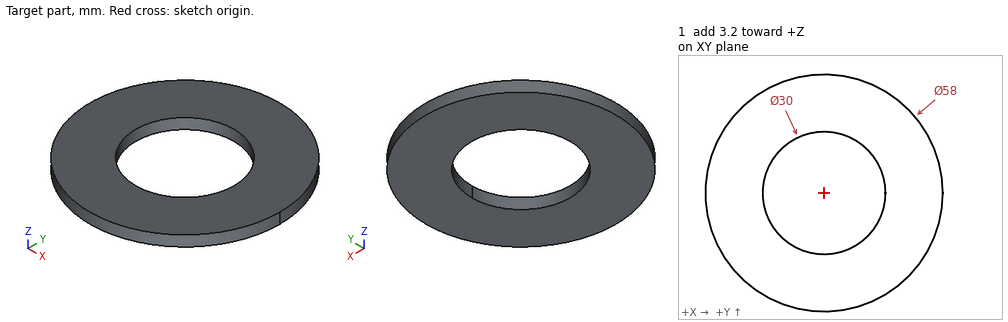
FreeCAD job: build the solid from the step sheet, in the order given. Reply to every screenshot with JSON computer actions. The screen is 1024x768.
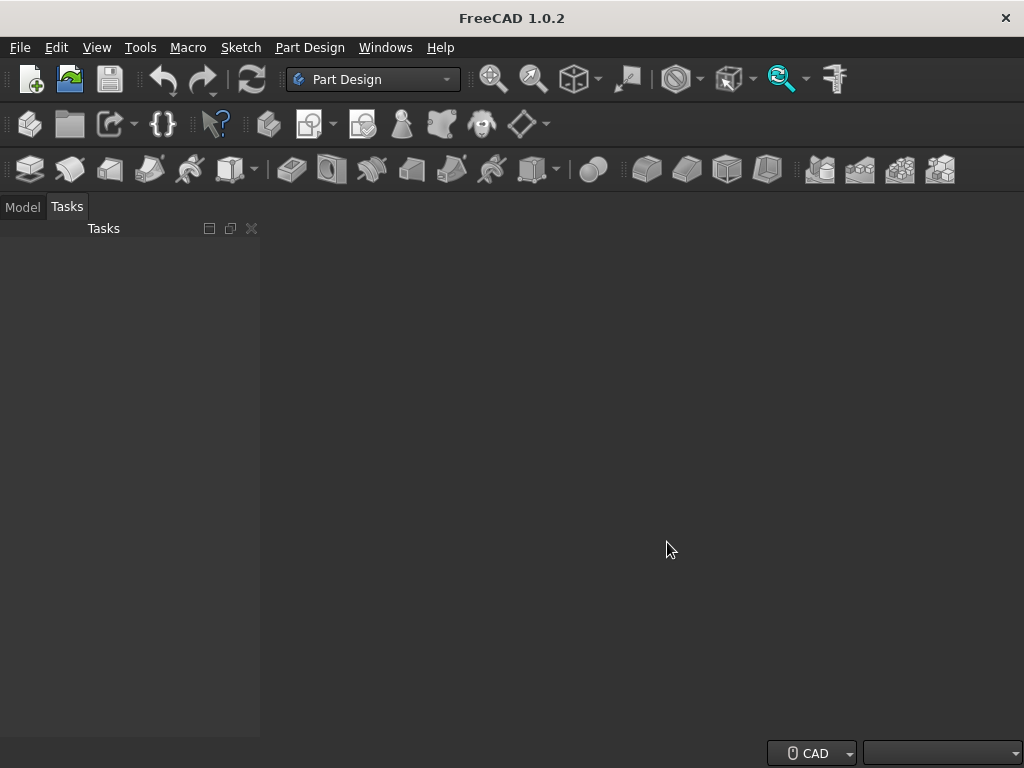
{"action": "left_click", "coordinate": [30, 80]}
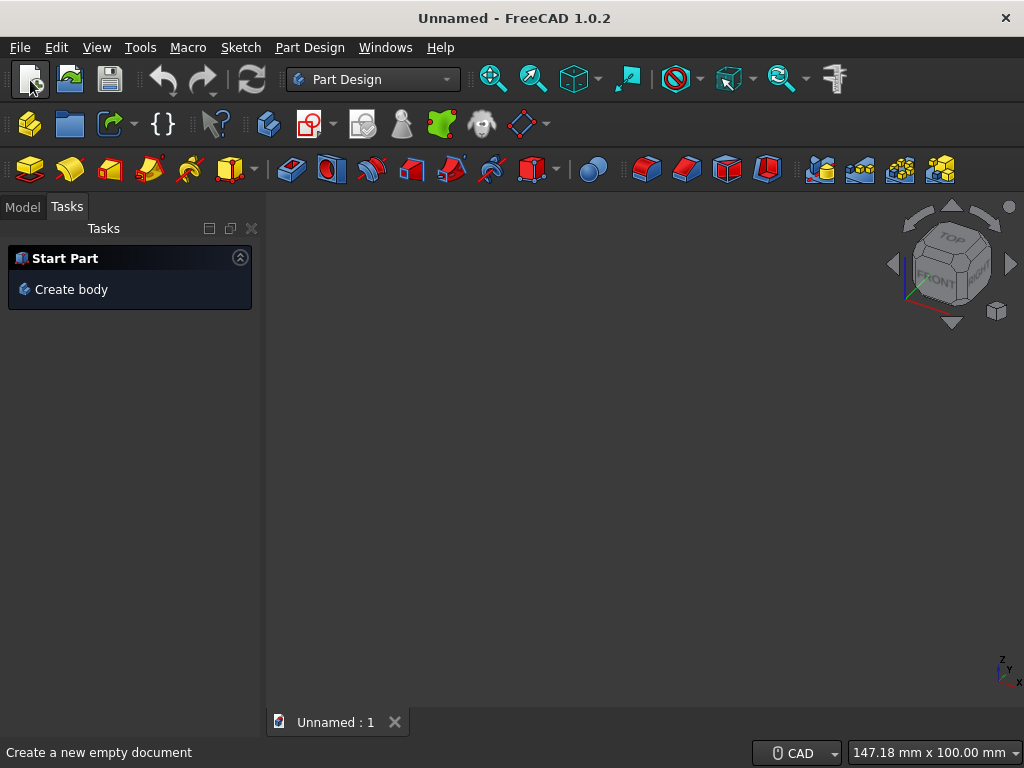
{"action": "left_click", "coordinate": [310, 124]}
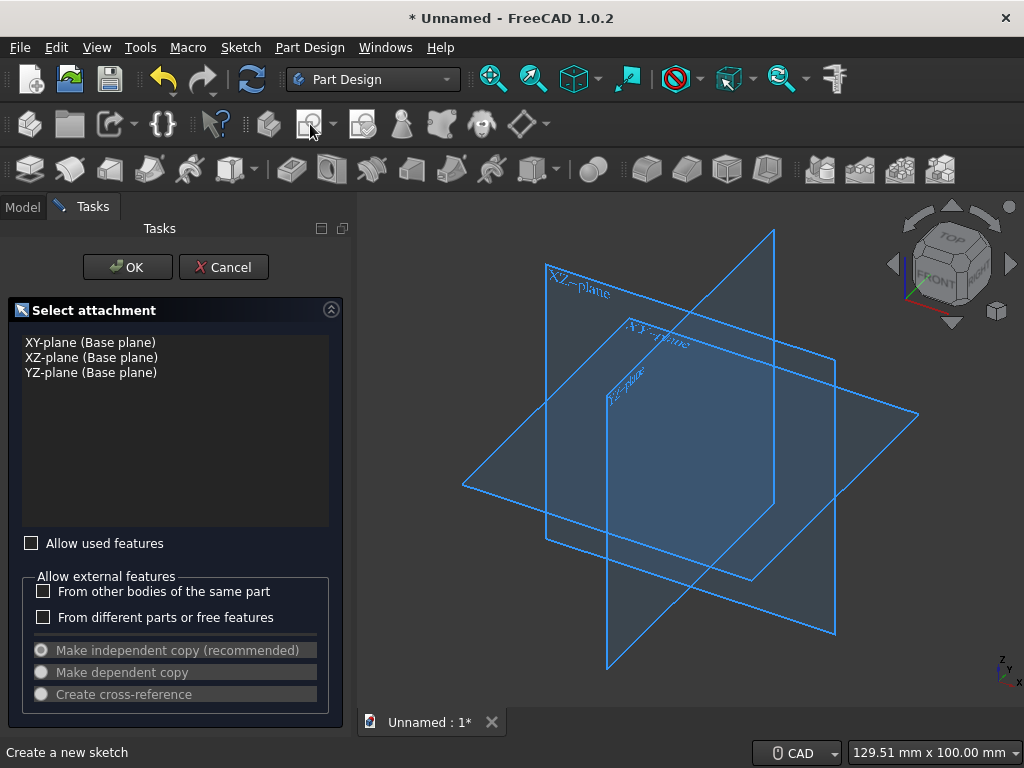
{"action": "left_click", "coordinate": [82, 342]}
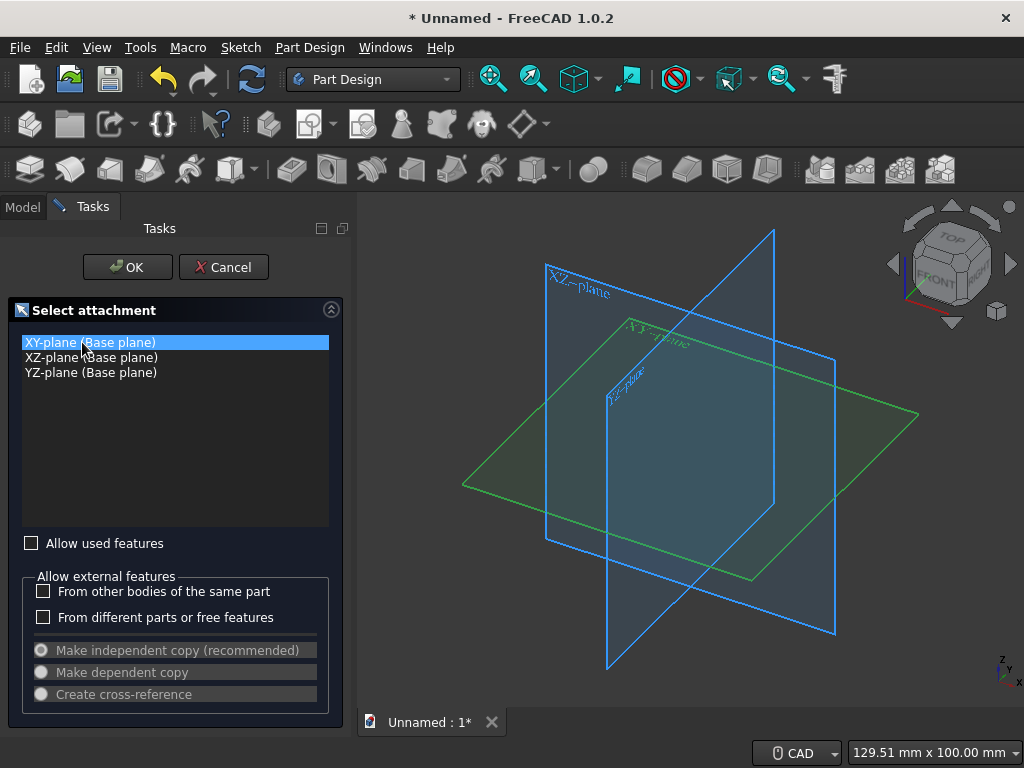
{"action": "left_click", "coordinate": [128, 267]}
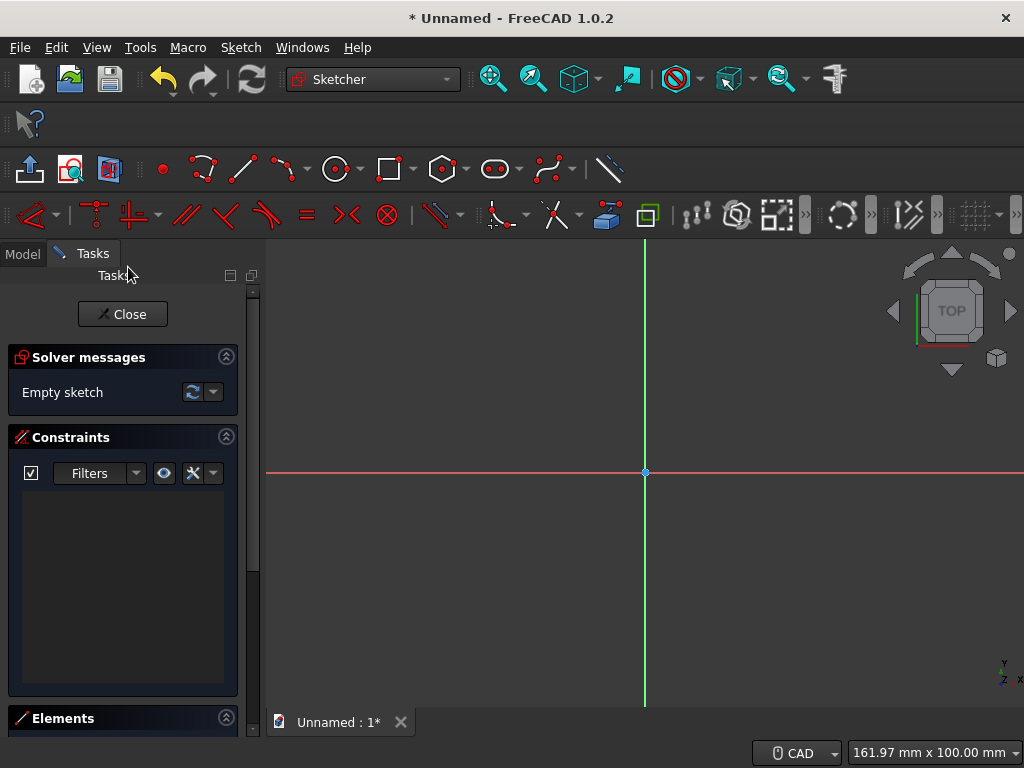
{"action": "left_click", "coordinate": [336, 170]}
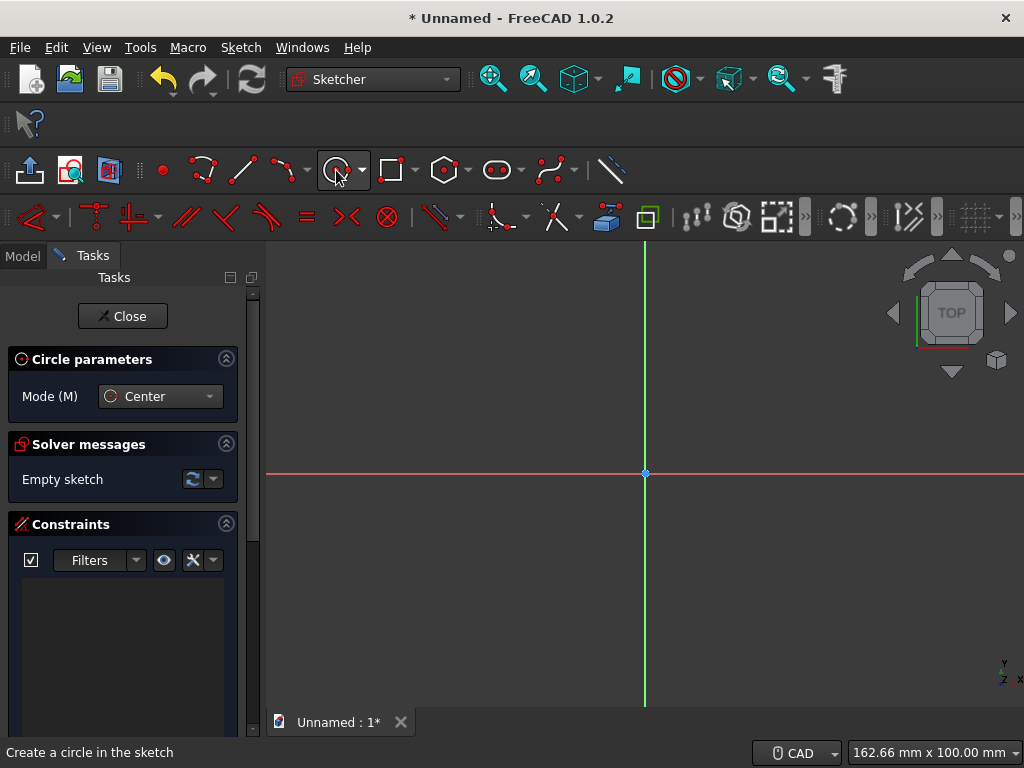
{"action": "left_click", "coordinate": [645, 474]}
{"action": "left_click", "coordinate": [741, 378]}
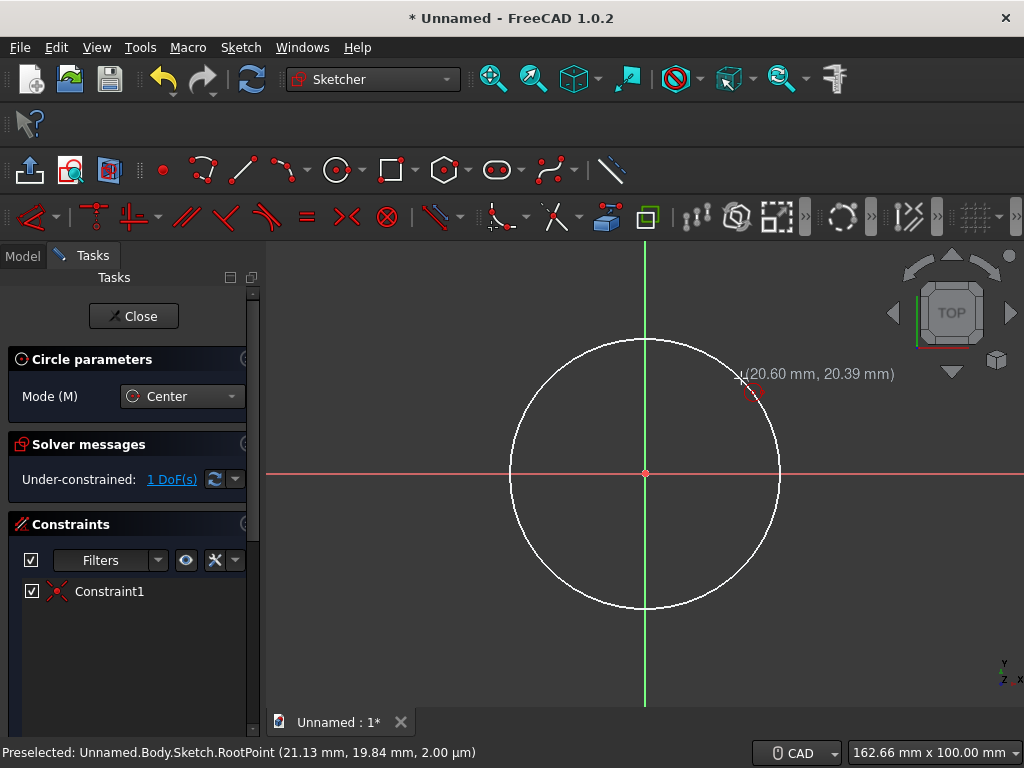
{"action": "left_click", "coordinate": [645, 474]}
{"action": "left_click", "coordinate": [694, 425]}
{"action": "key", "text": "Escape"}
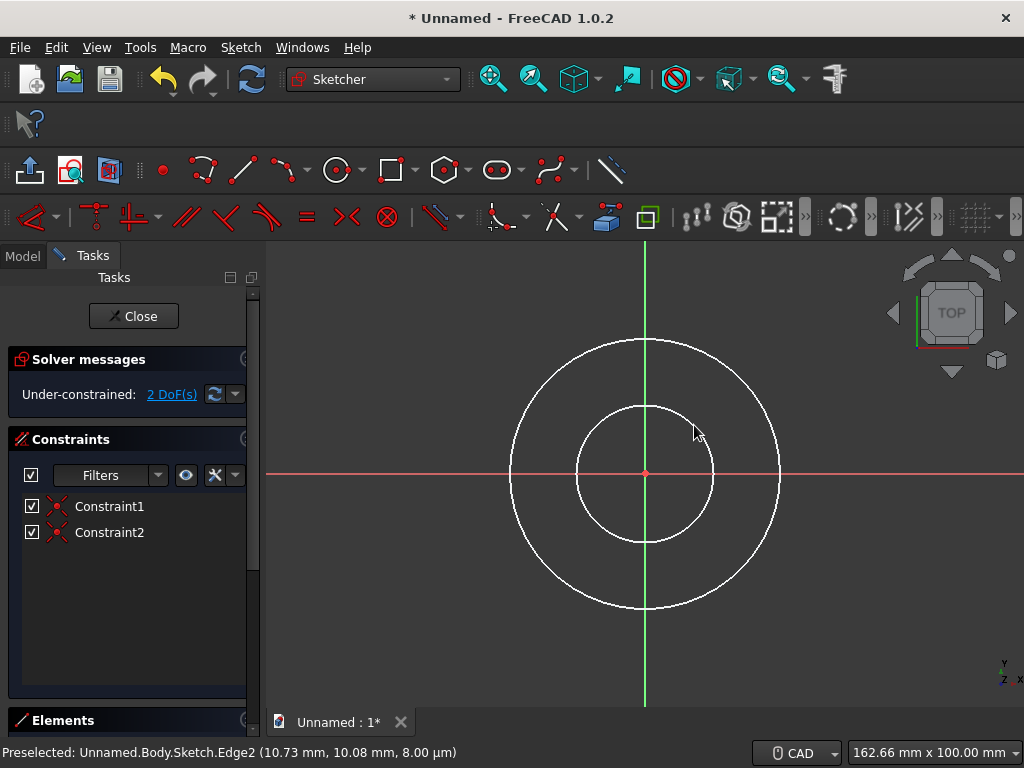
{"action": "left_click", "coordinate": [32, 218]}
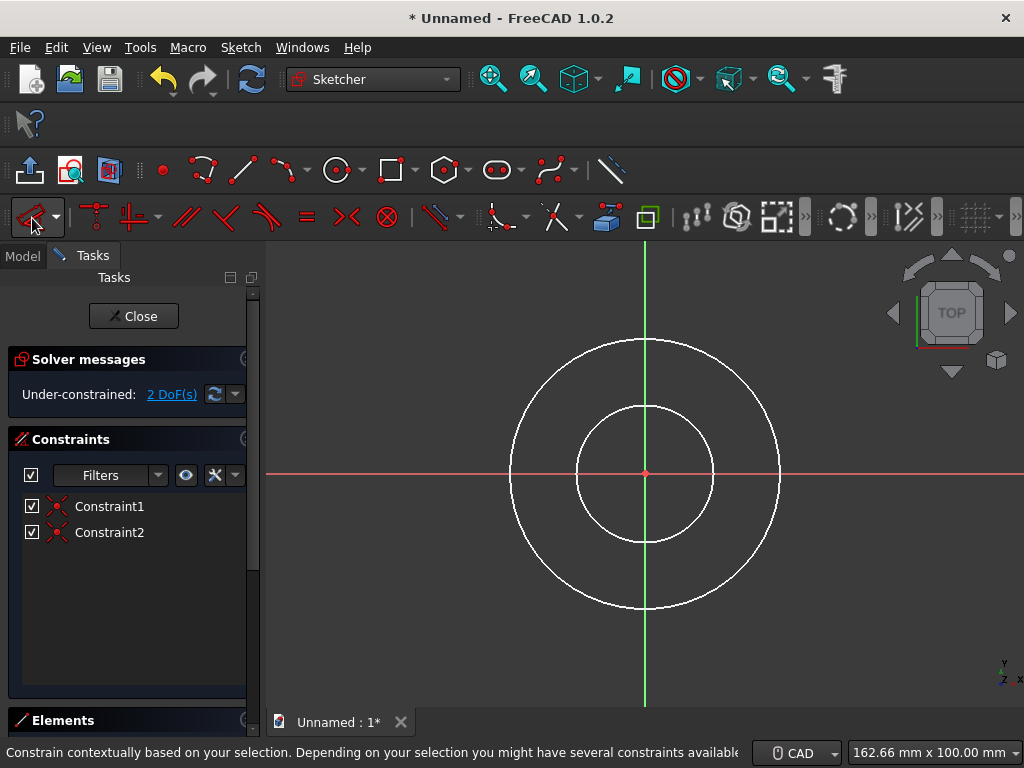
{"action": "left_click", "coordinate": [740, 378]}
{"action": "left_click", "coordinate": [763, 355]}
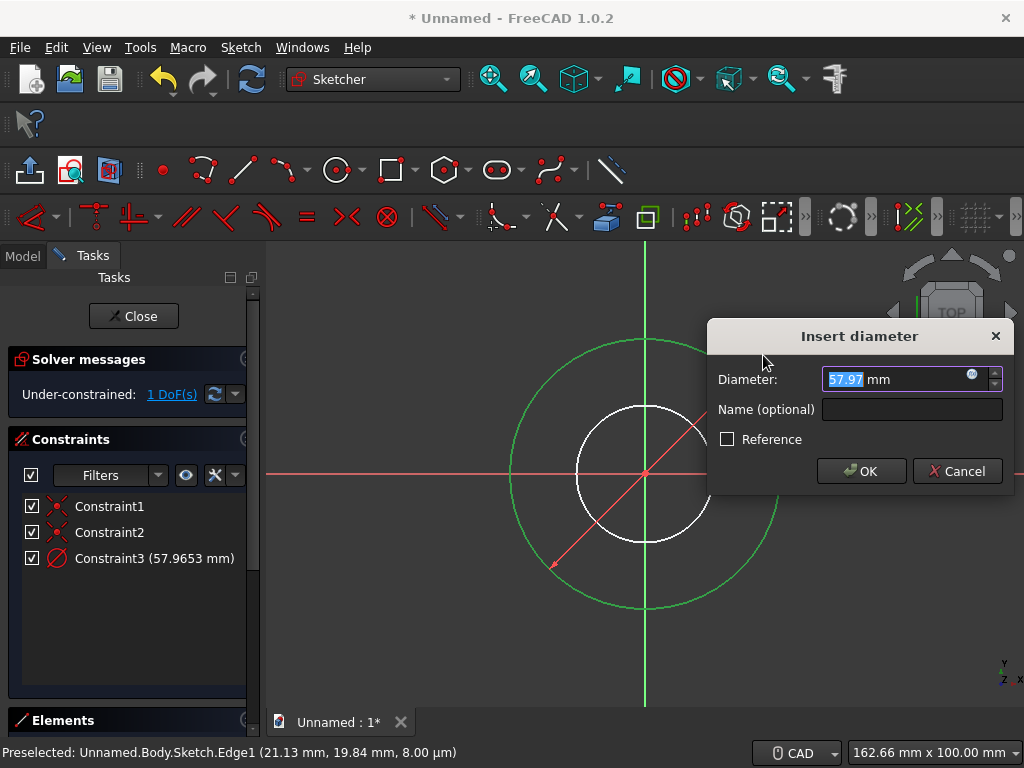
{"action": "type", "text": "58"}
{"action": "key", "text": "Return"}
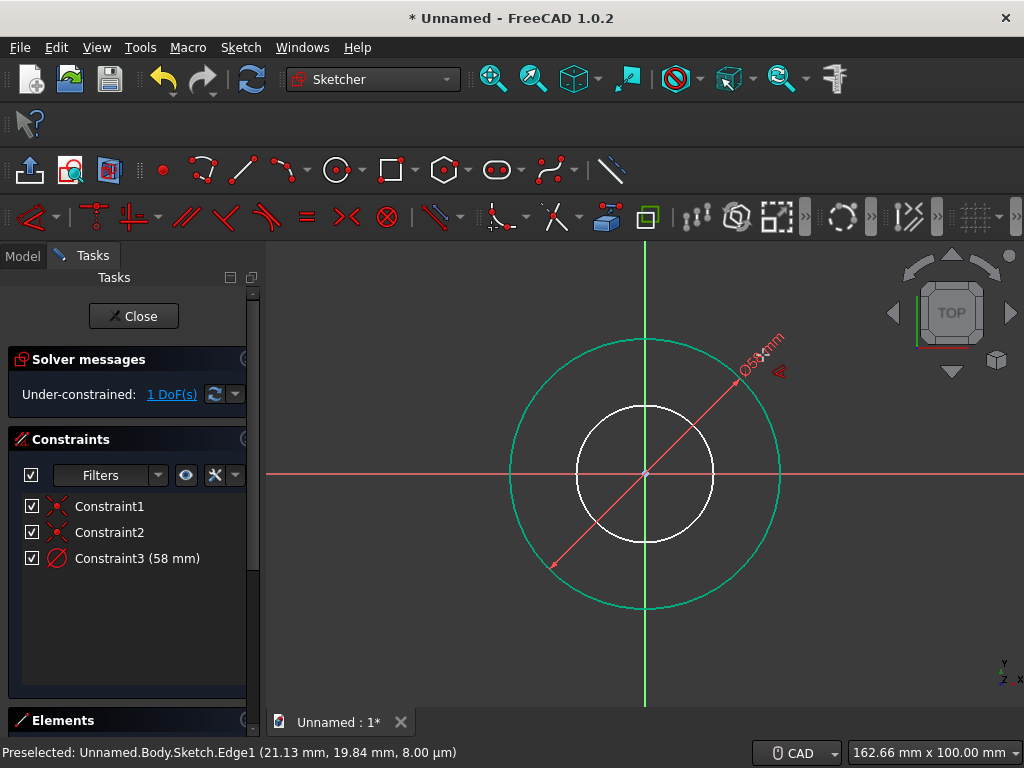
{"action": "left_click", "coordinate": [693, 425]}
{"action": "left_click", "coordinate": [715, 402]}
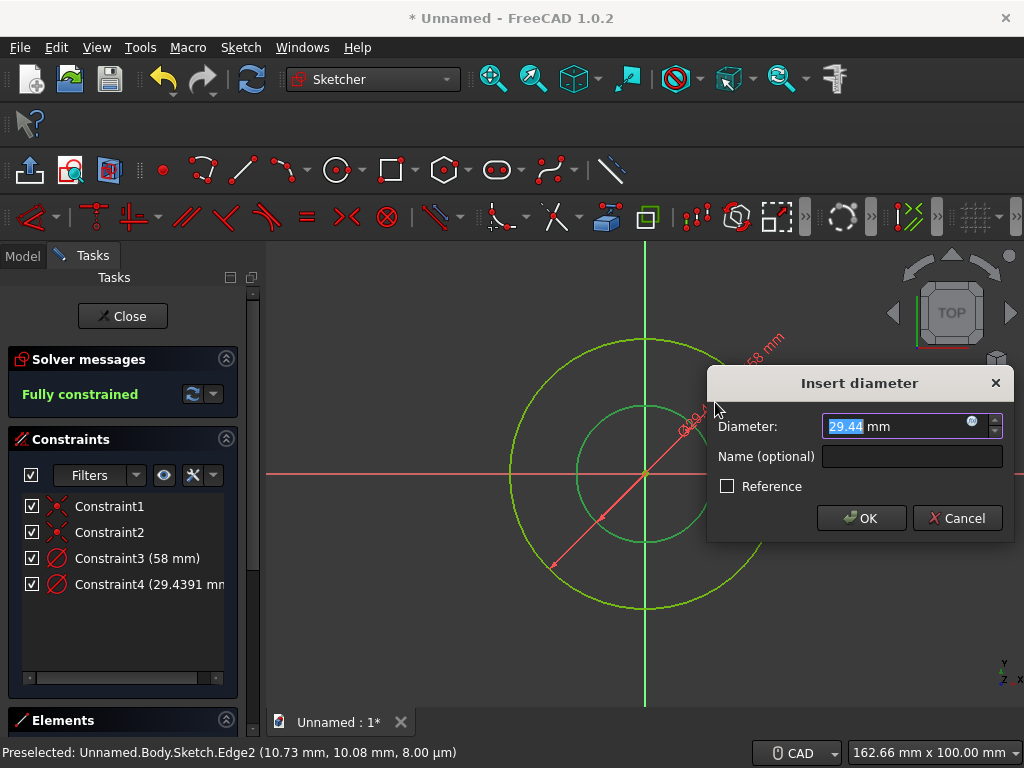
{"action": "type", "text": "30"}
{"action": "key", "text": "Return"}
{"action": "key", "text": "Escape"}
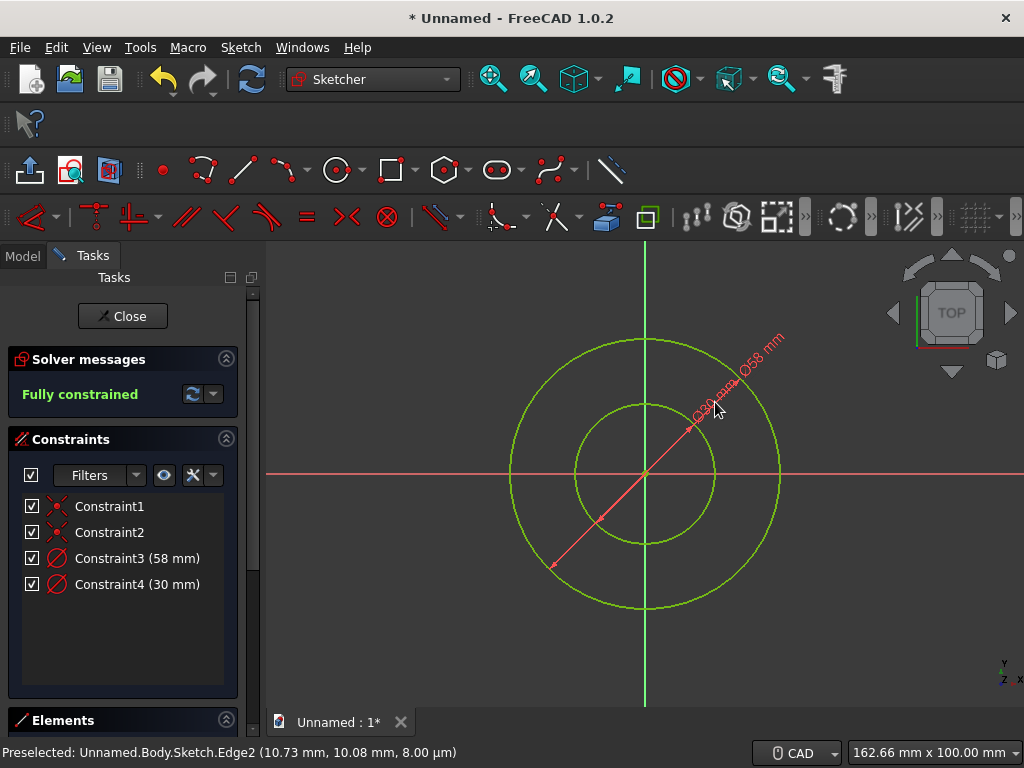
{"action": "left_click", "coordinate": [123, 316]}